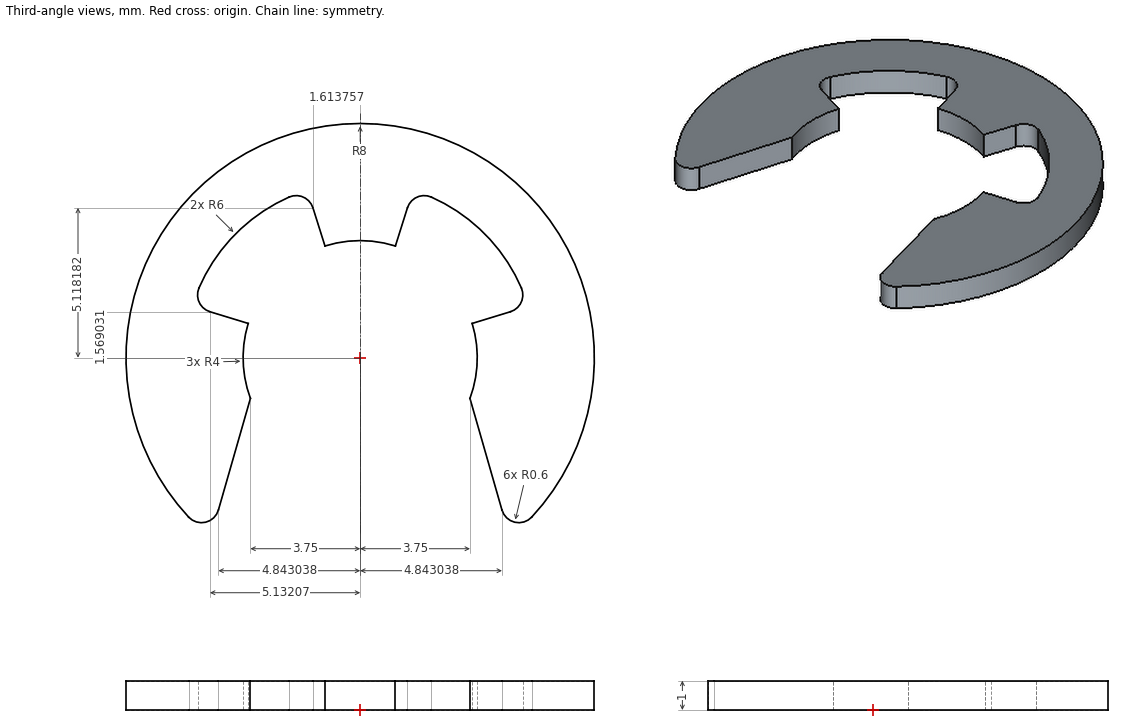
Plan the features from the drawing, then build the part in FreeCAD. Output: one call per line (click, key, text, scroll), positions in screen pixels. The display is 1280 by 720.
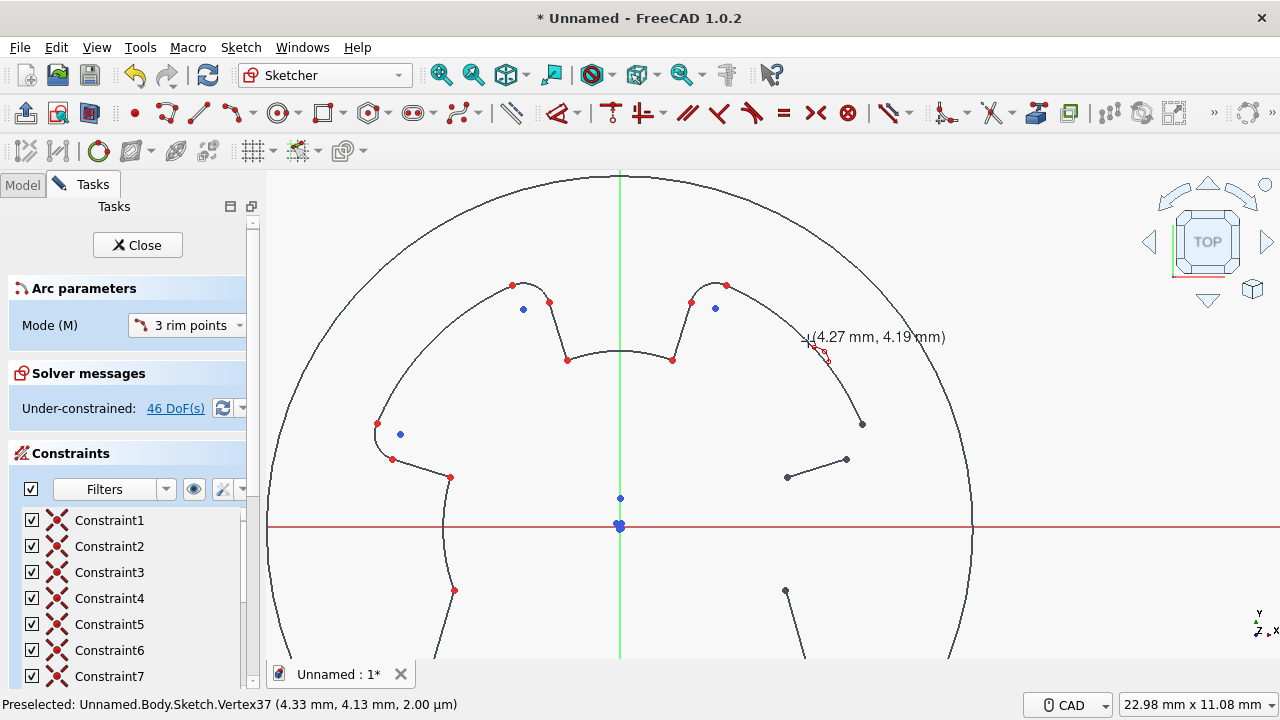
click(862, 425)
click(846, 459)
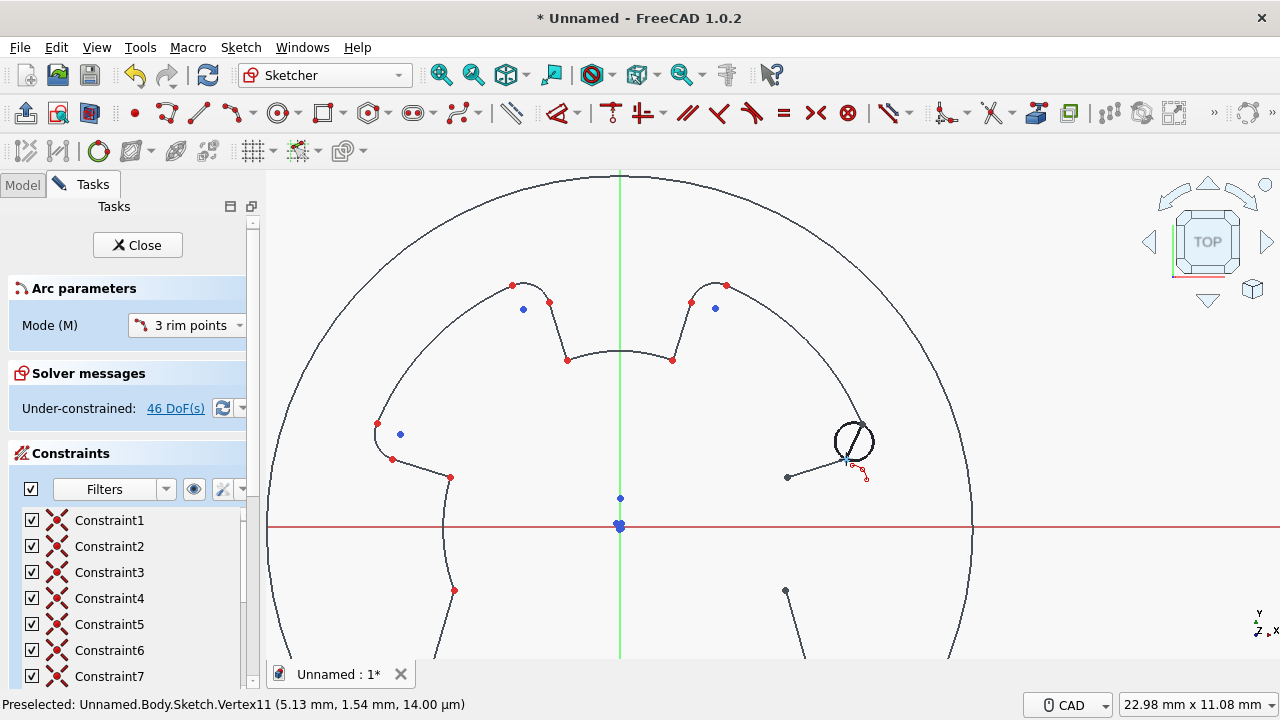
scroll(862, 444, up, 3)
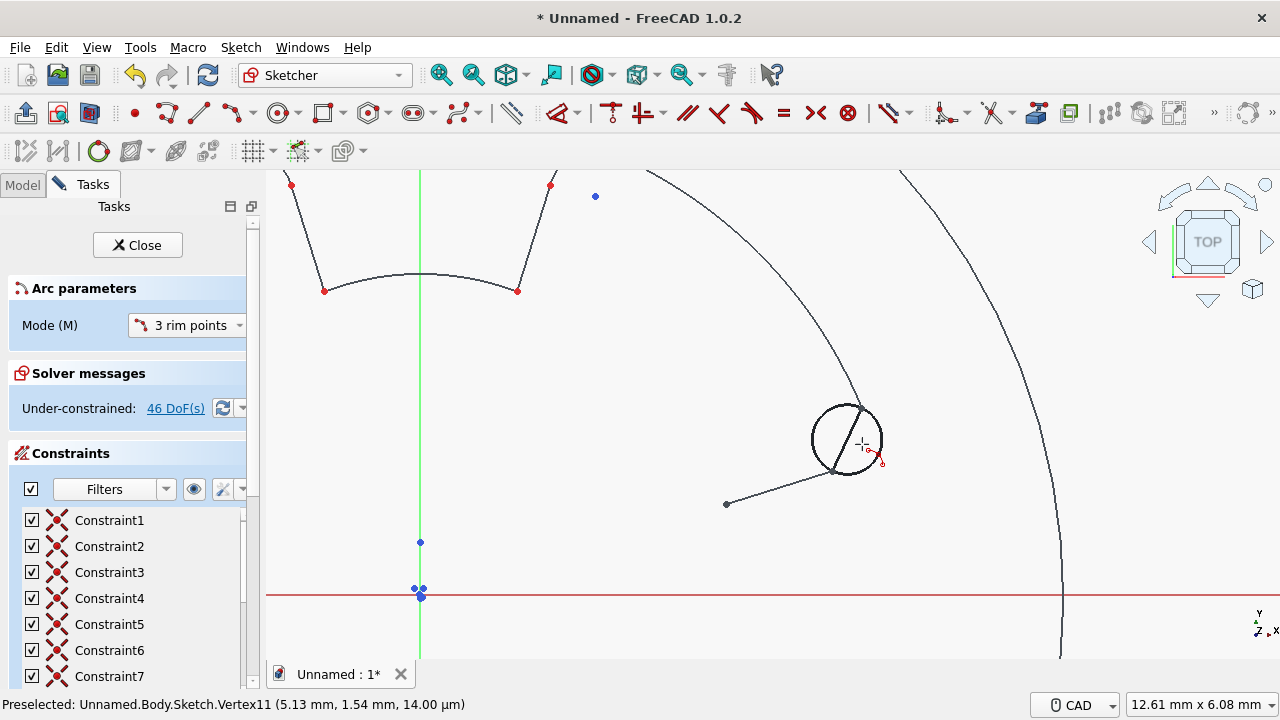
click(862, 443)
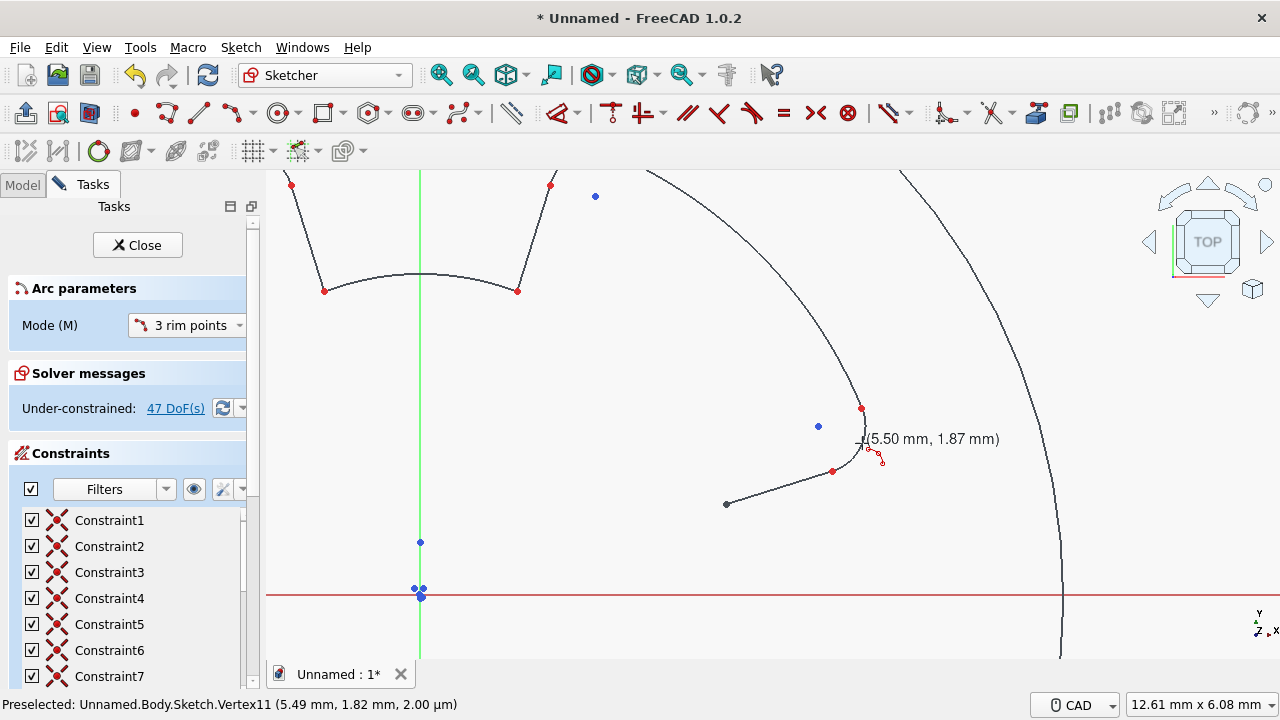
click(726, 504)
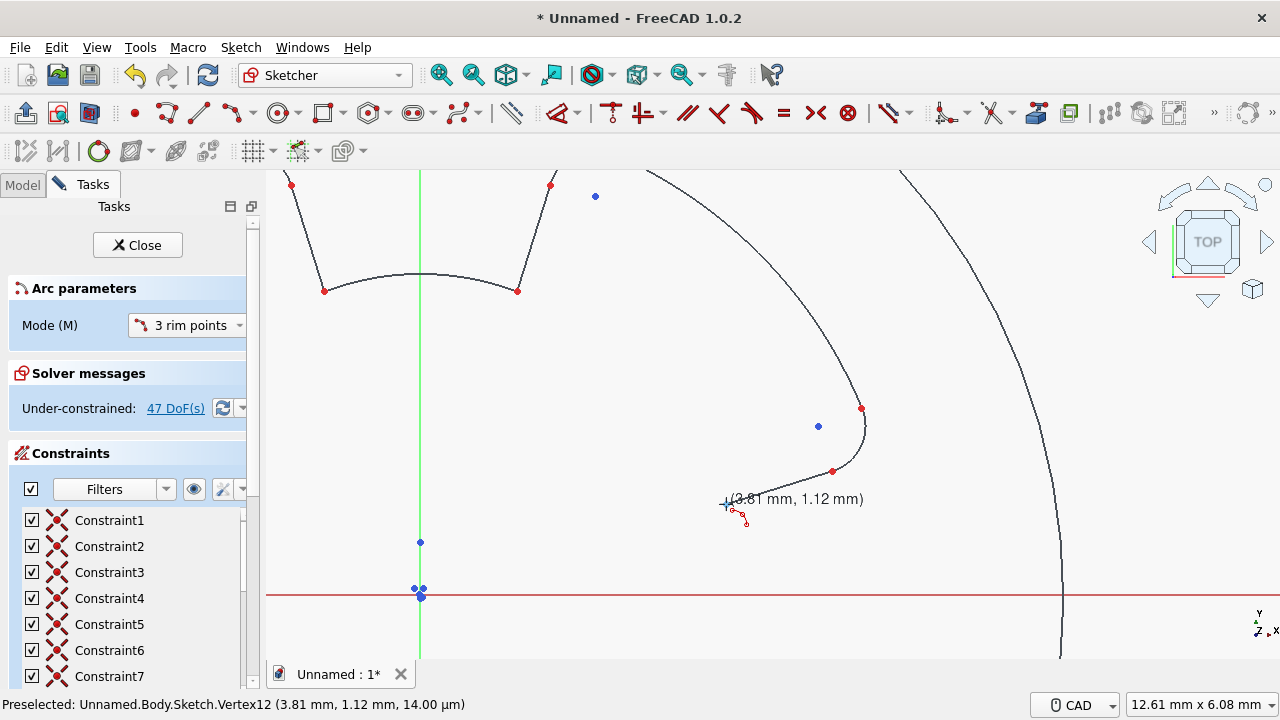
scroll(827, 378, down, 6)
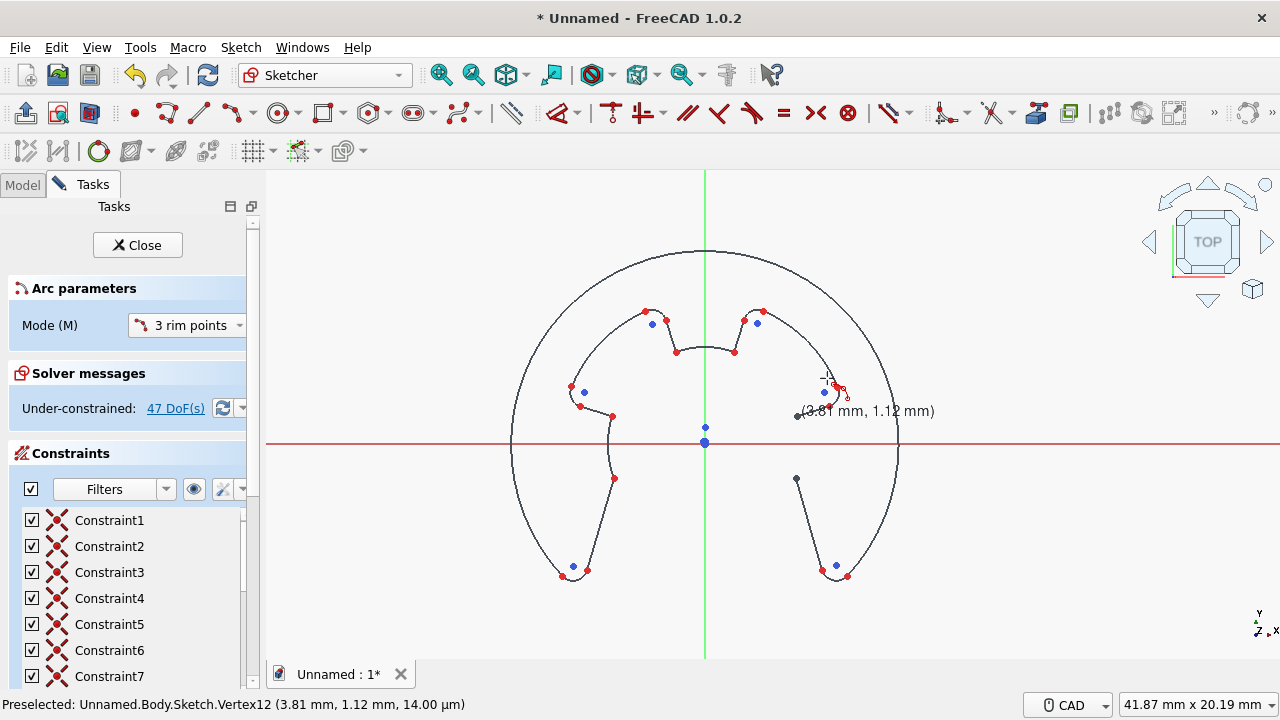
click(796, 478)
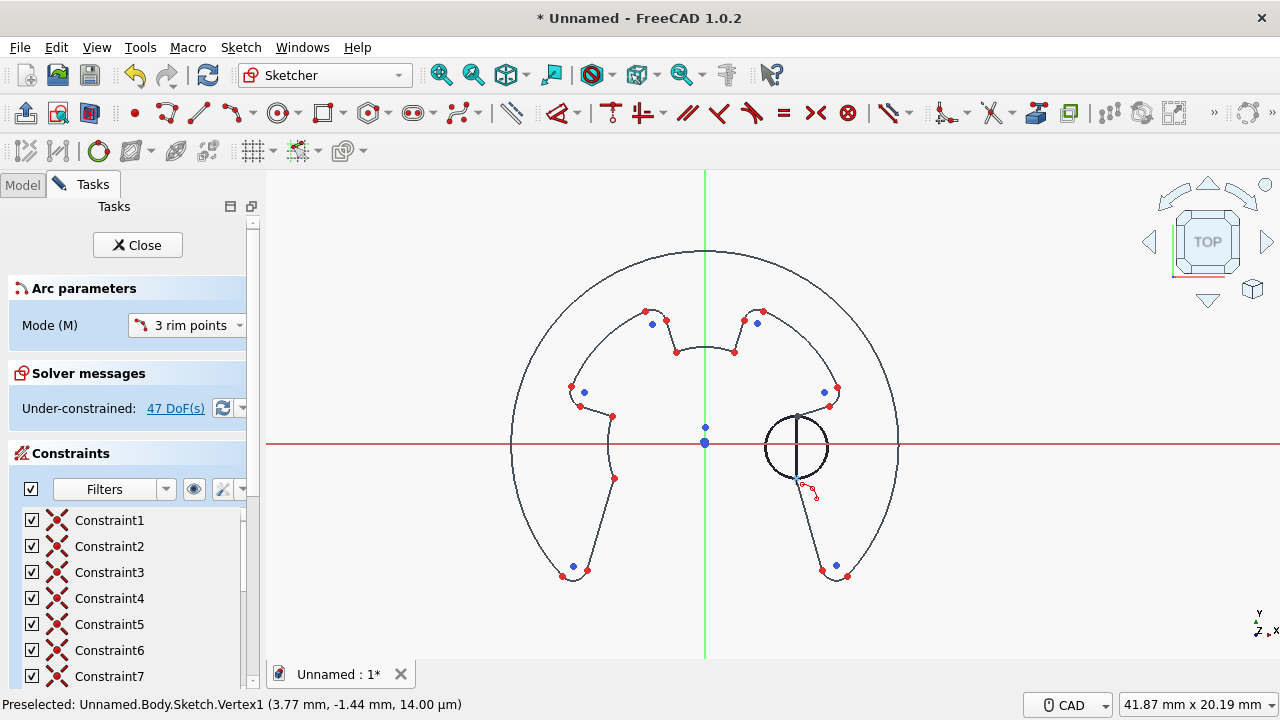
scroll(801, 453, up, 6)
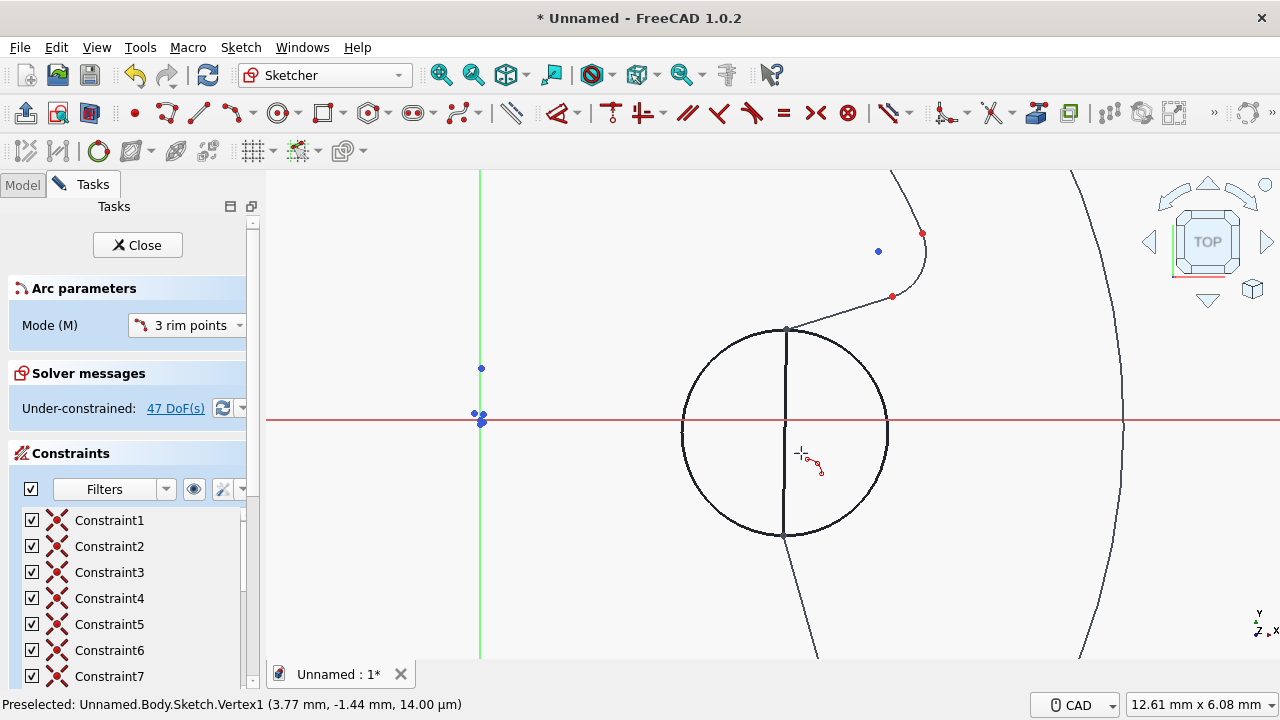
click(801, 451)
key(Escape)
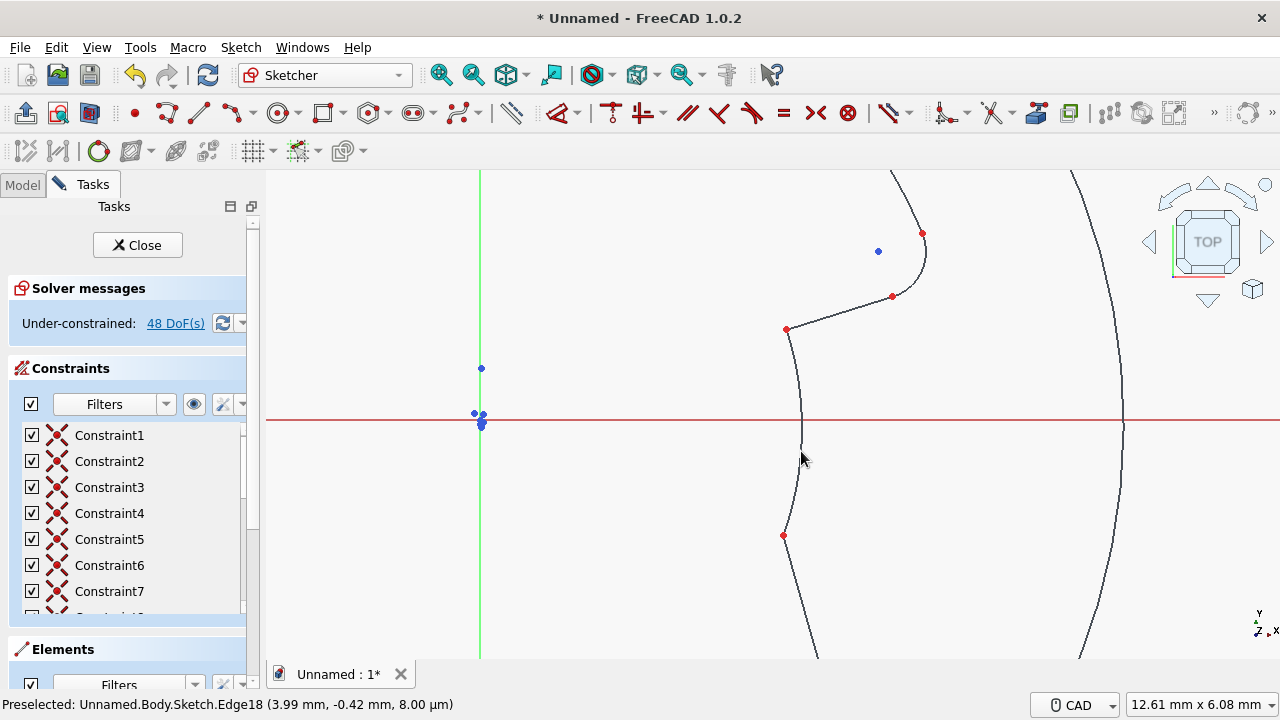
click(809, 627)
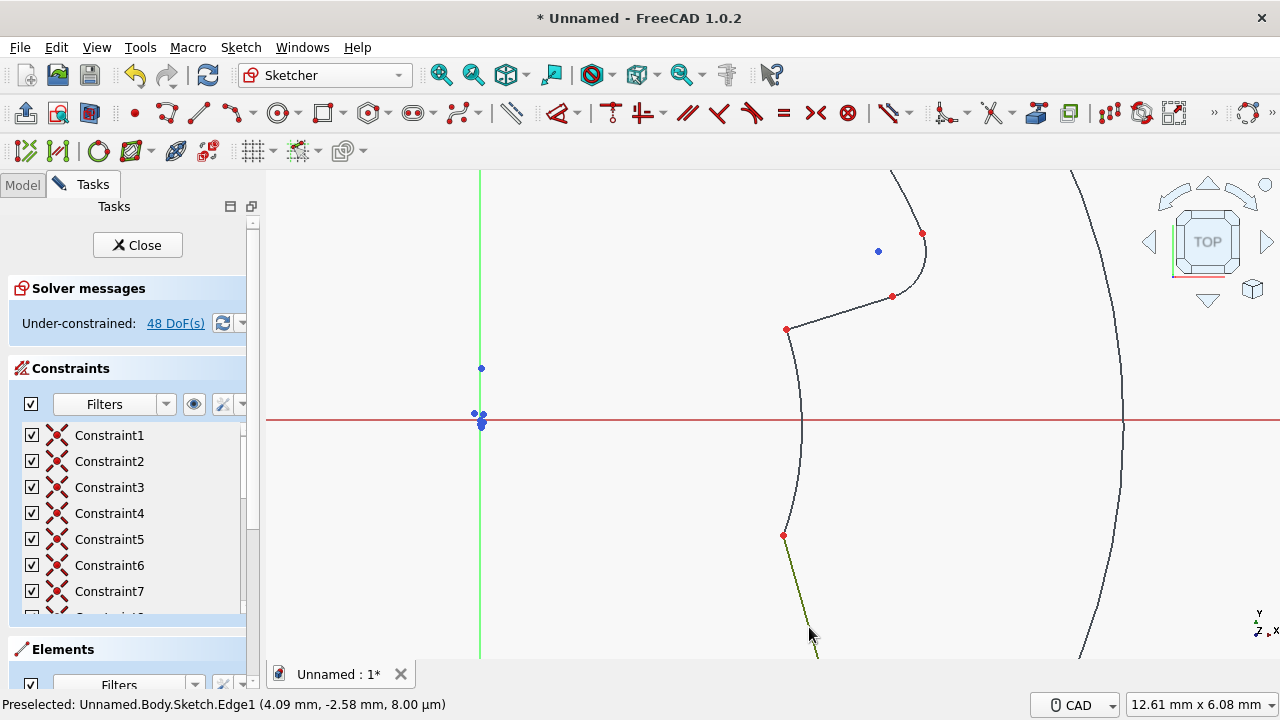
scroll(801, 453, down, 6)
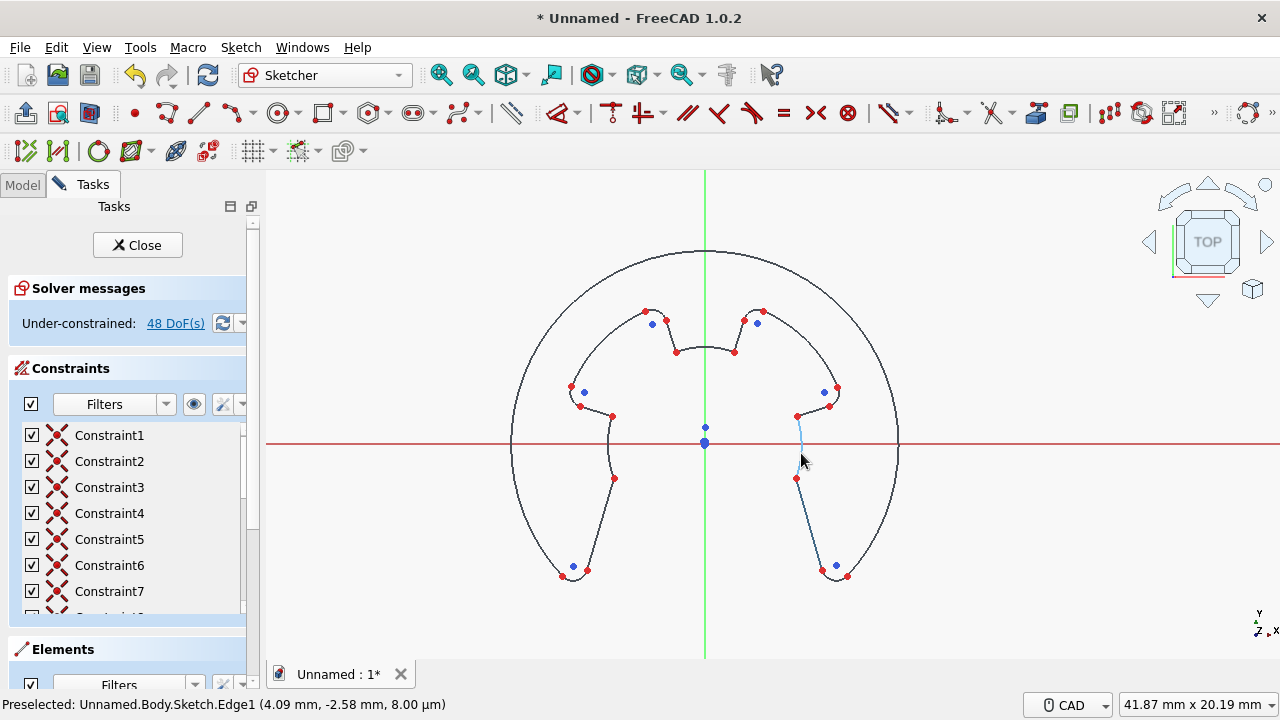
scroll(827, 578, up, 3)